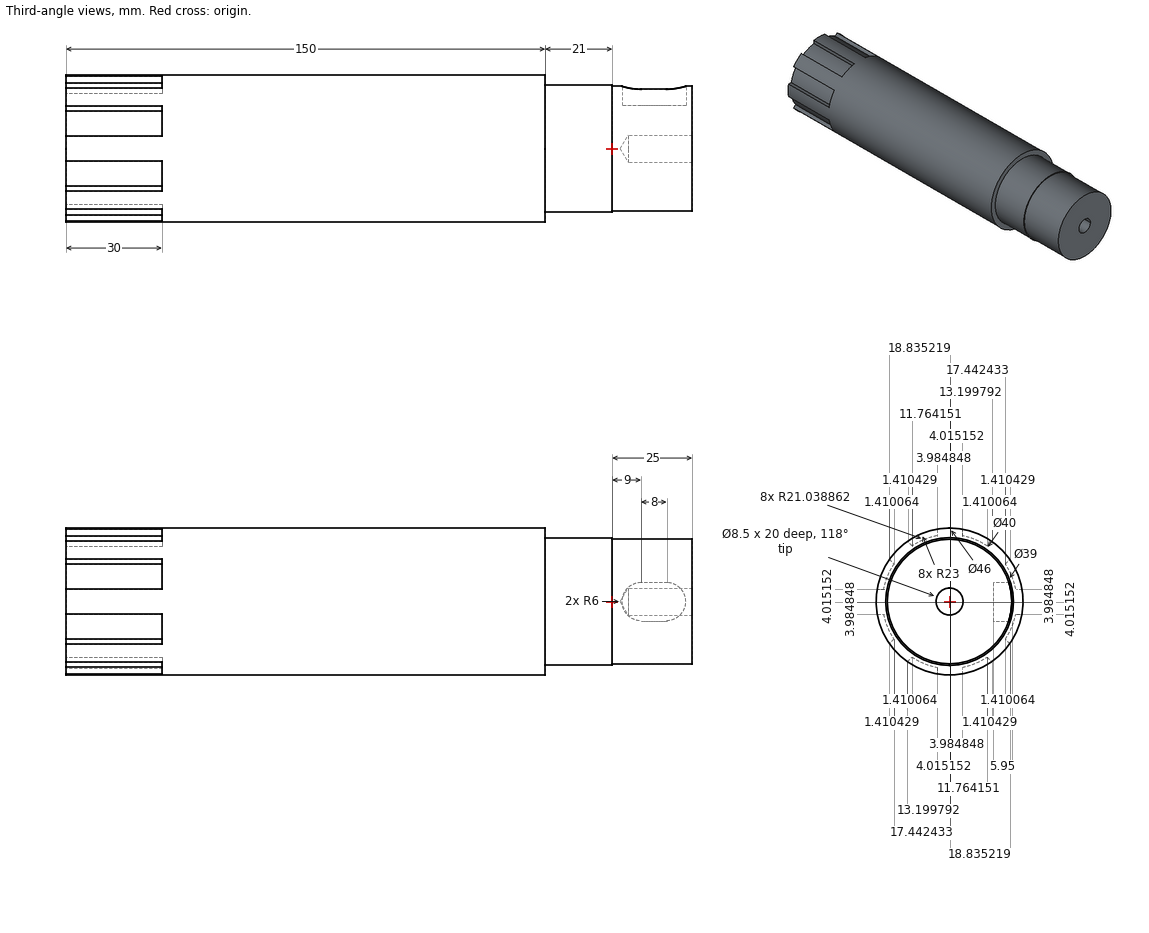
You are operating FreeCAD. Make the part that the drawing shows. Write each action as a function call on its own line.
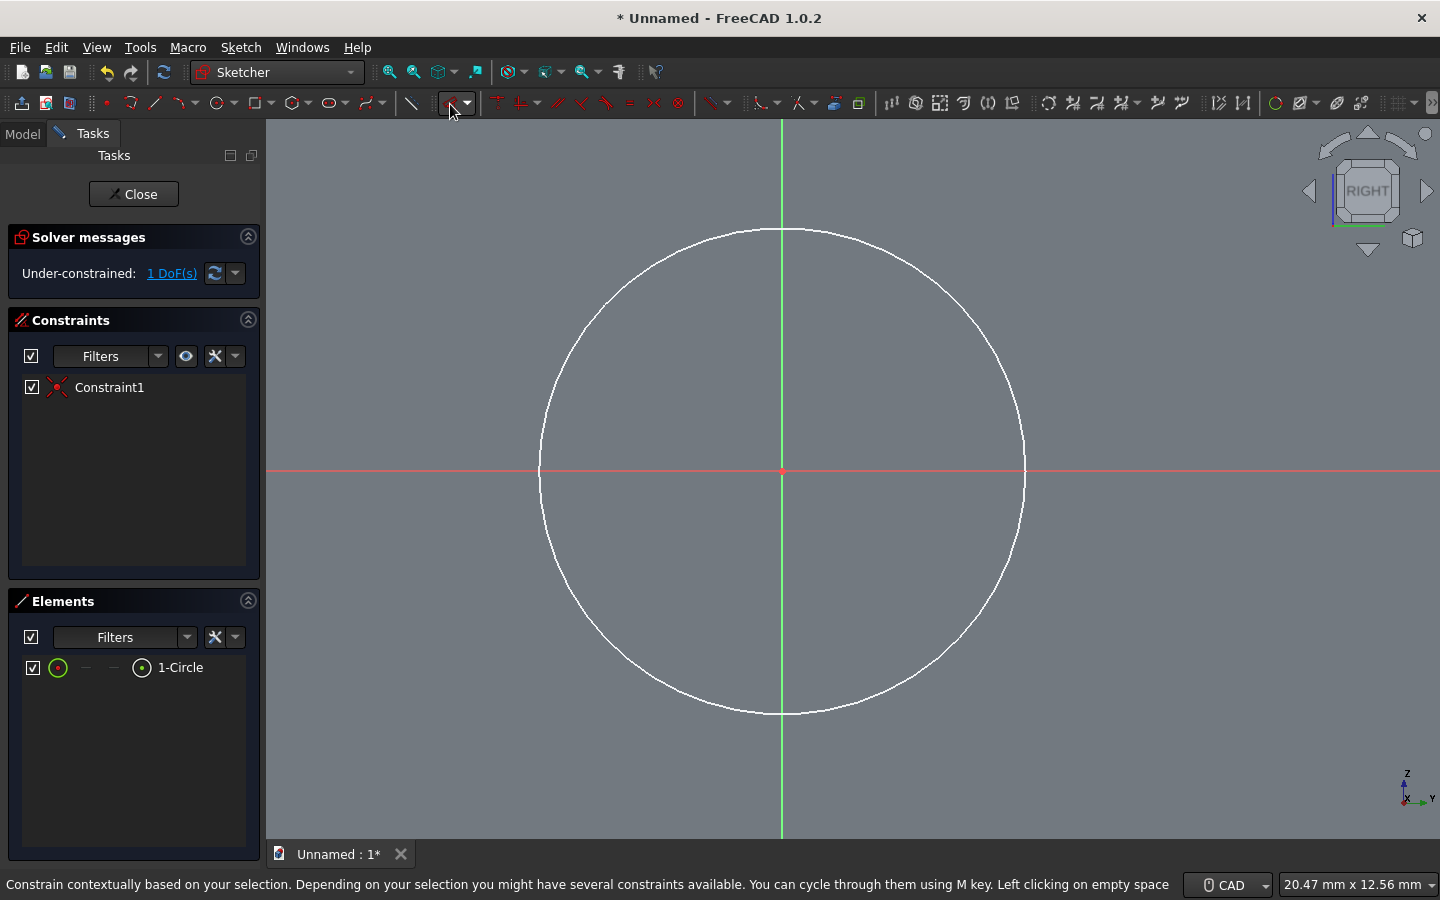
click(954, 299)
click(977, 276)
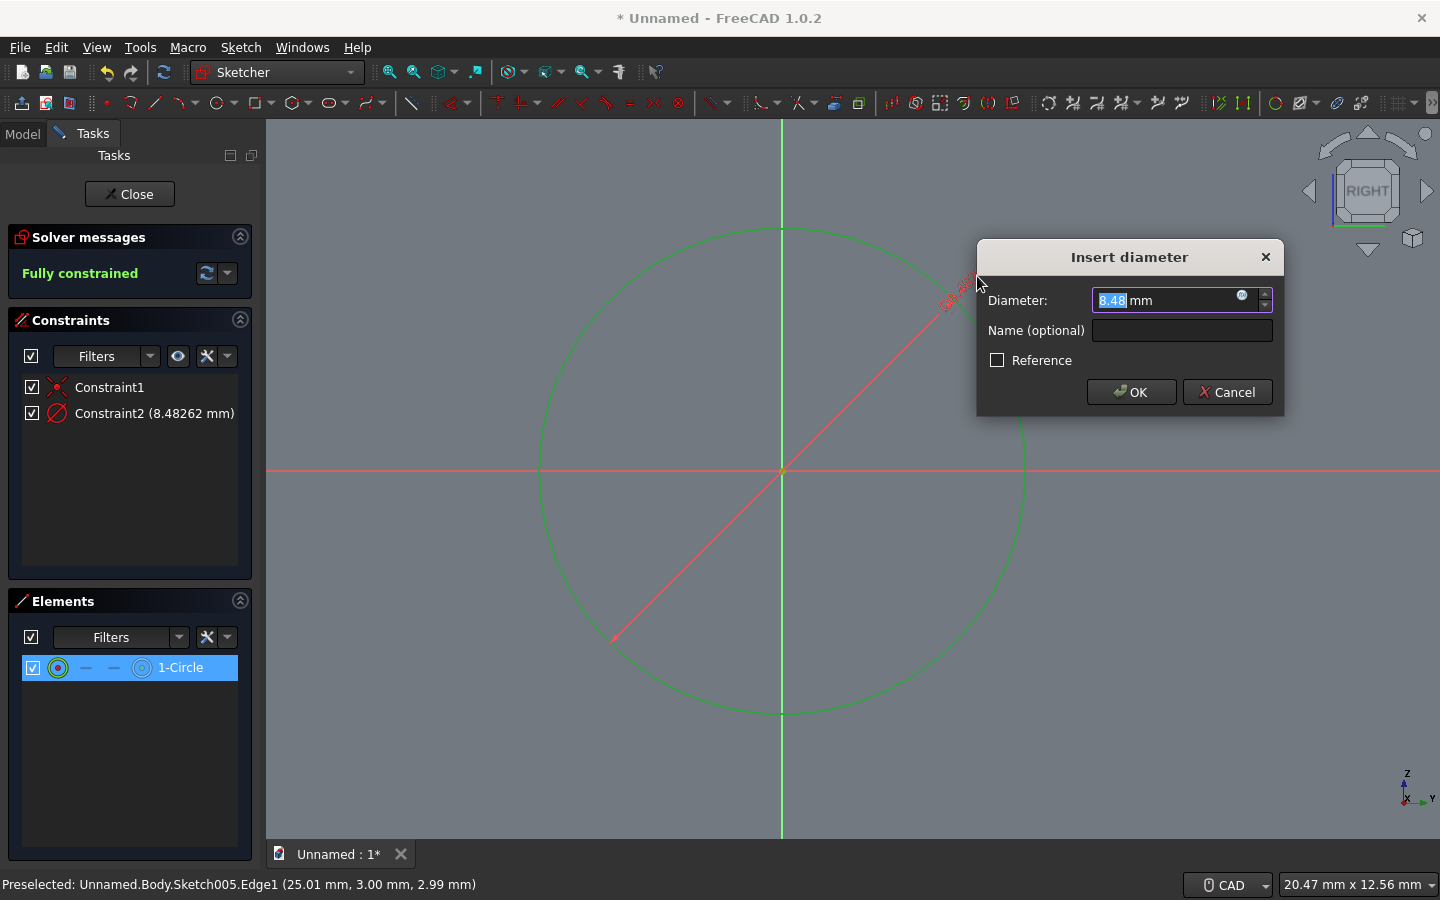
text(8.5)
key(Return)
key(Escape)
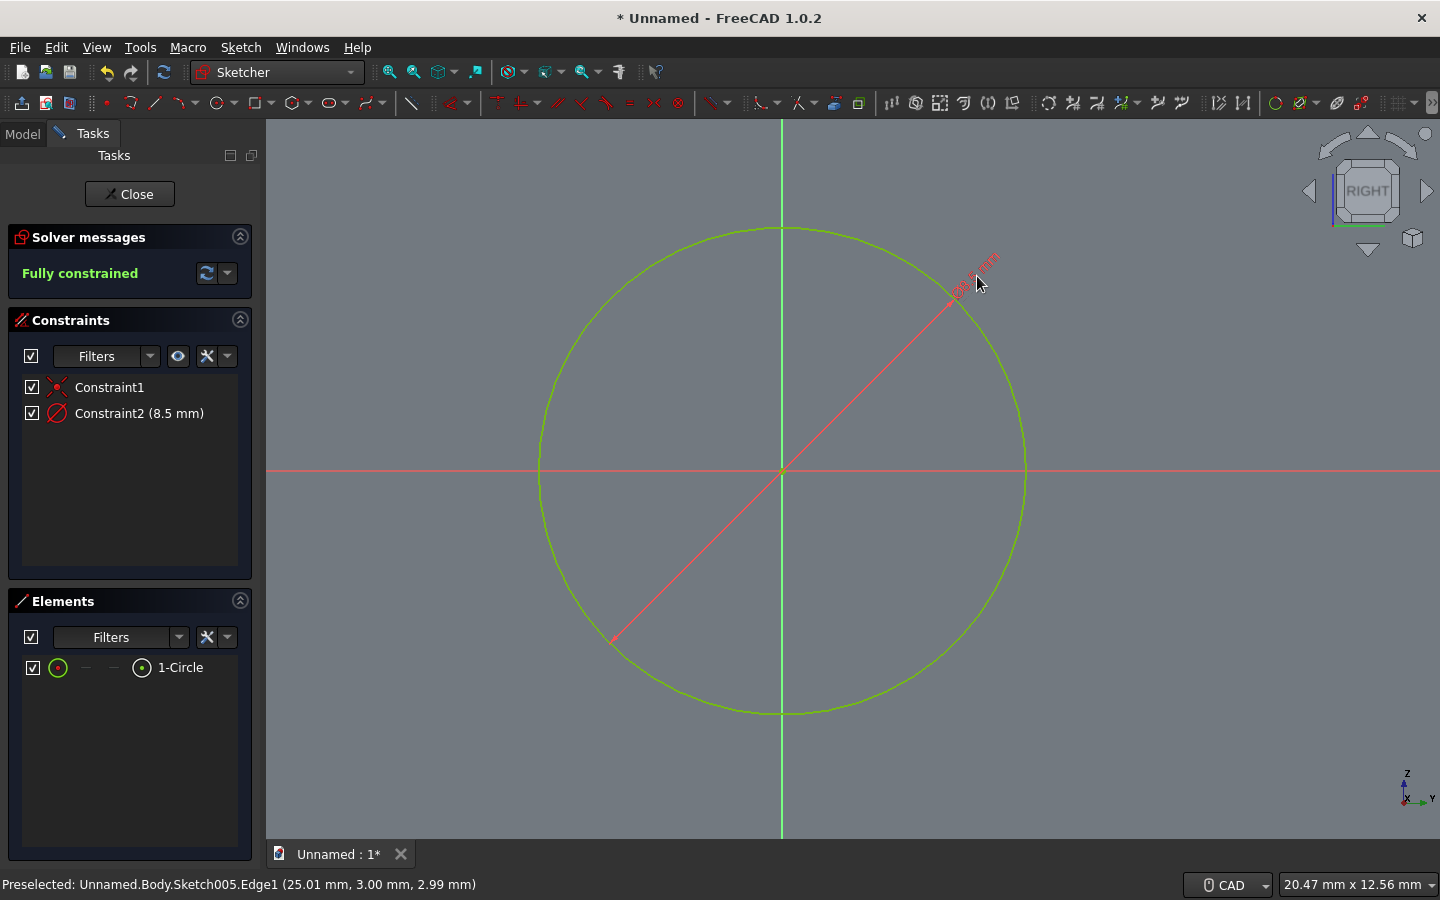
click(130, 194)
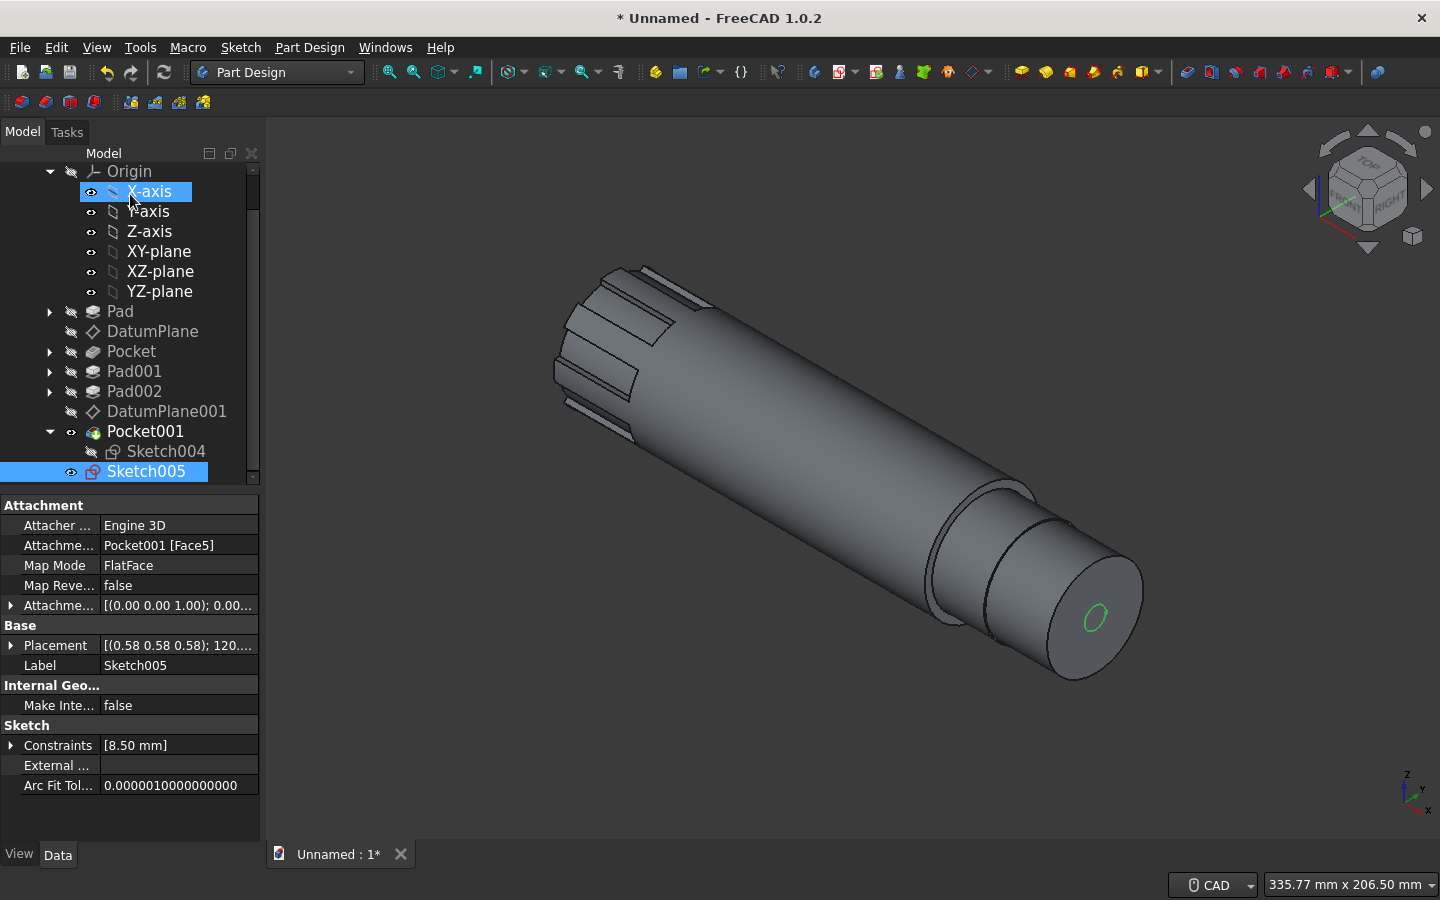
click(1212, 72)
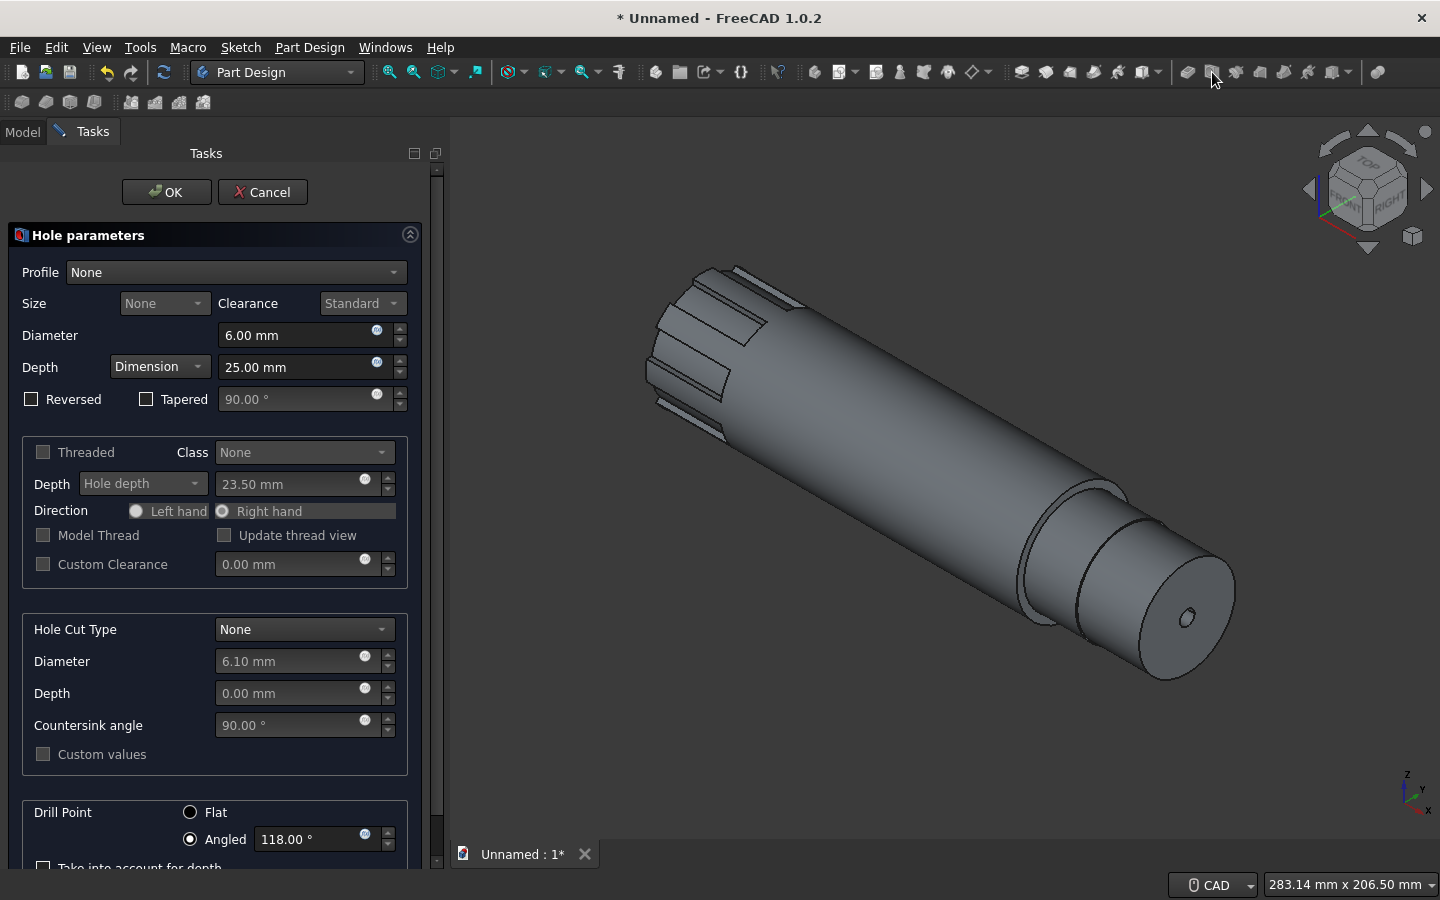
triple_click(305, 335)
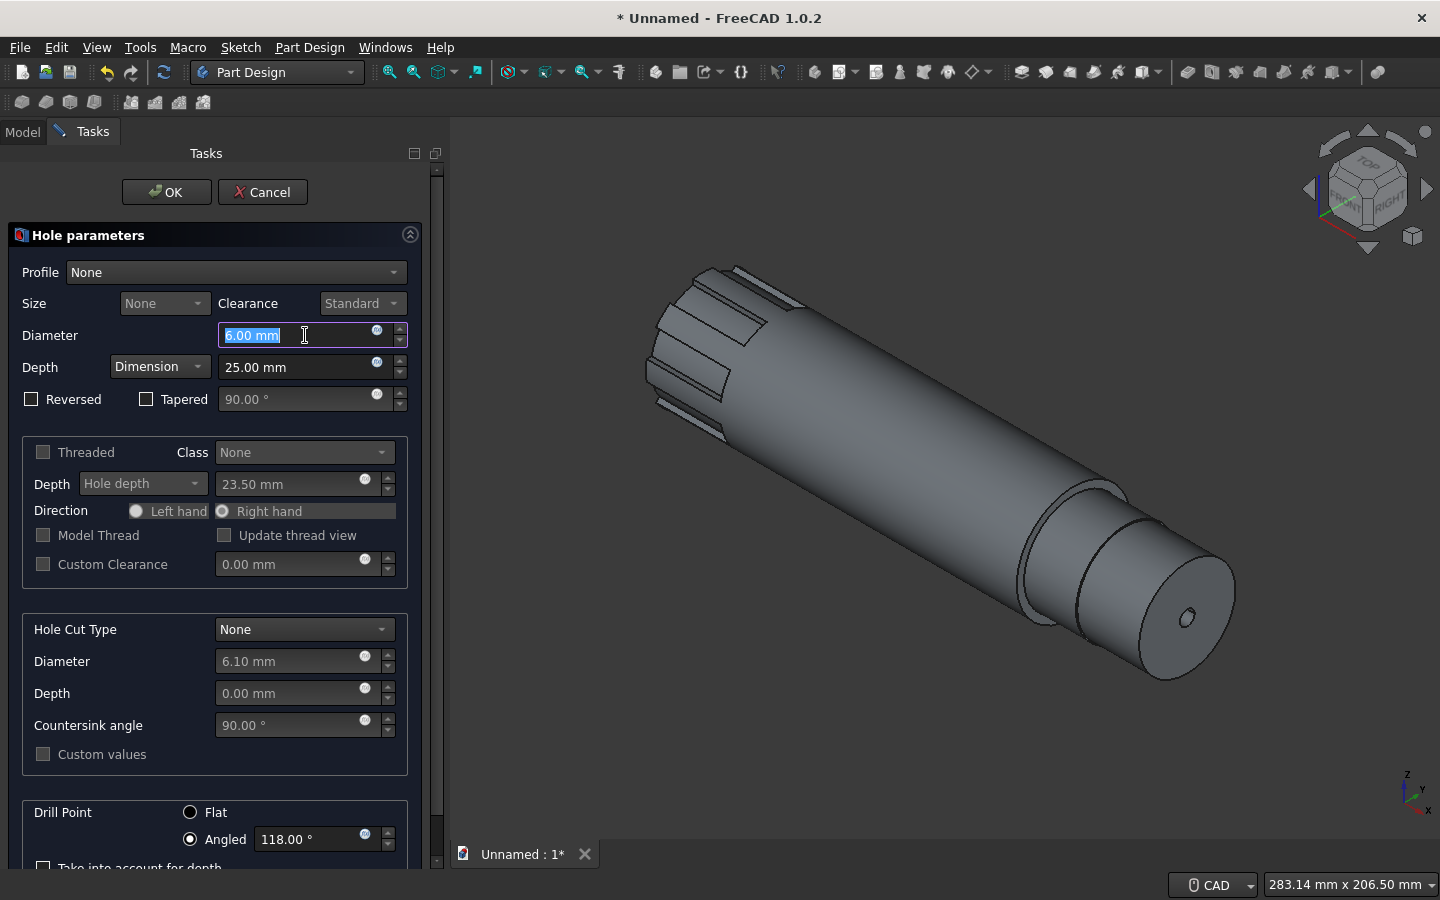
text(8.5)
key(Tab)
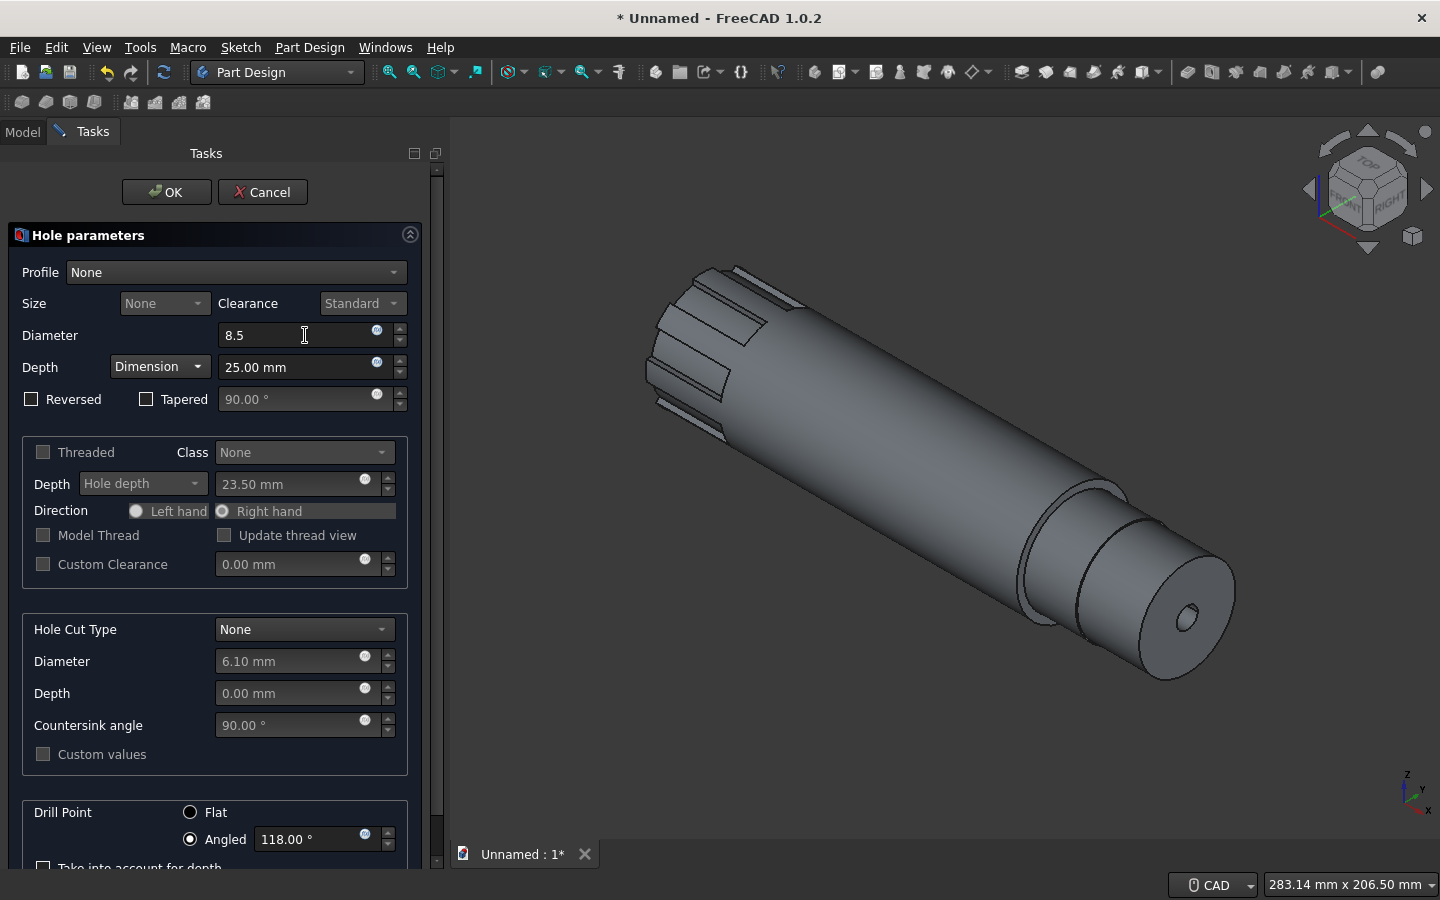
triple_click(305, 367)